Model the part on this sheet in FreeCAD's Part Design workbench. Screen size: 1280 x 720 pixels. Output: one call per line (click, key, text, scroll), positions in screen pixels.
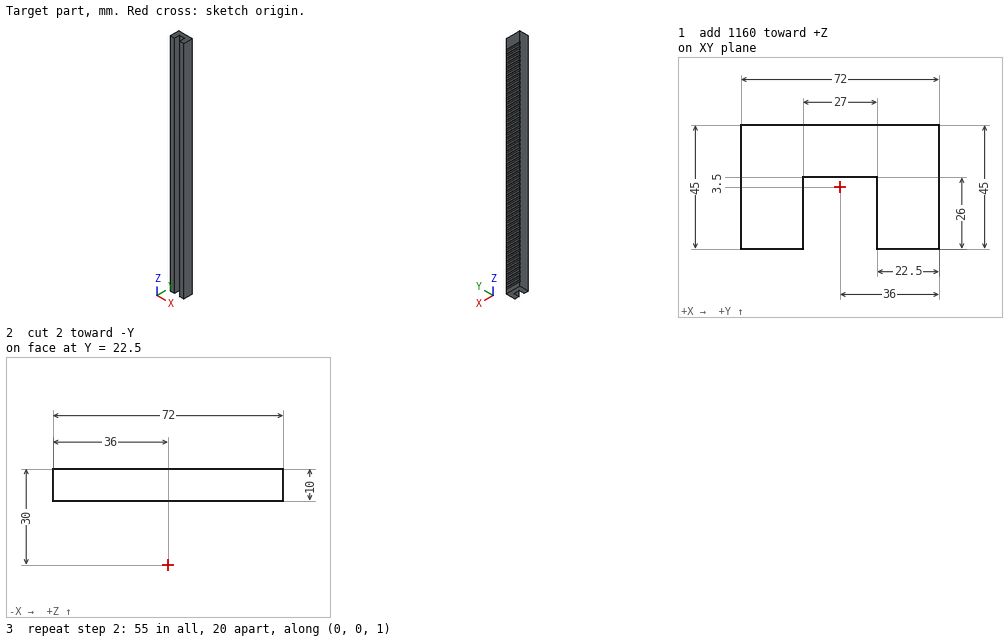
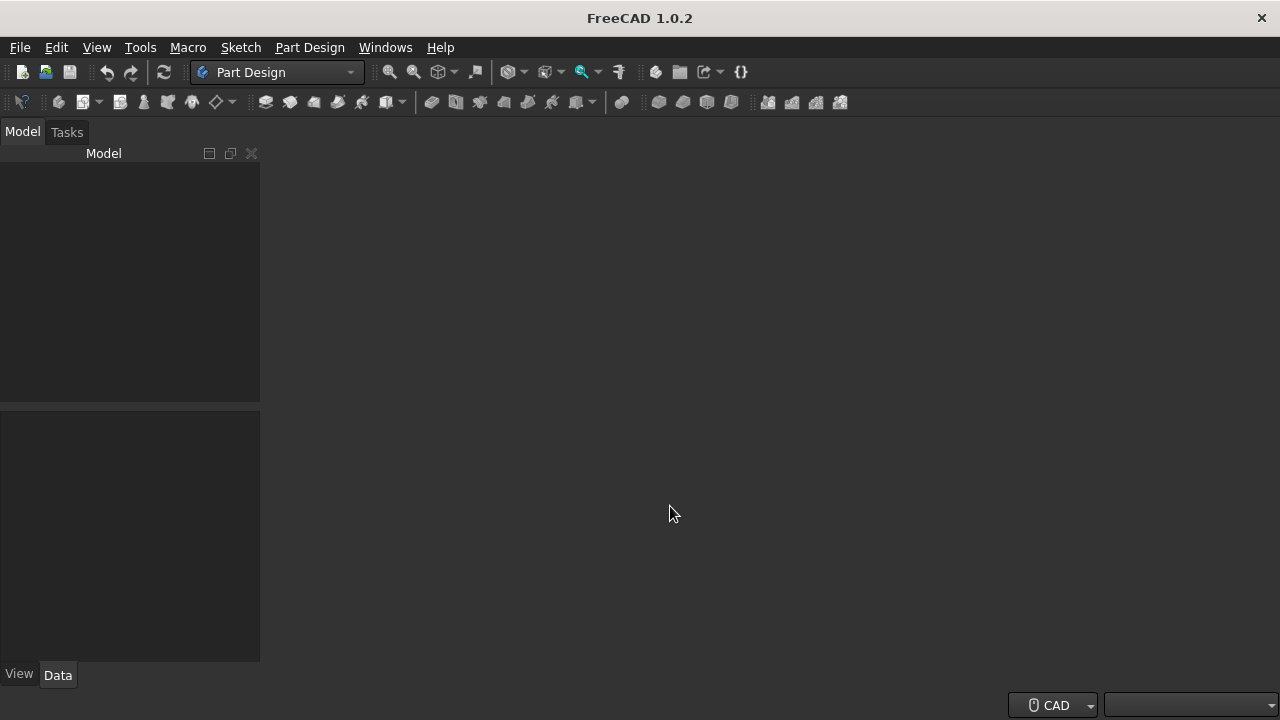
key(ctrl+n)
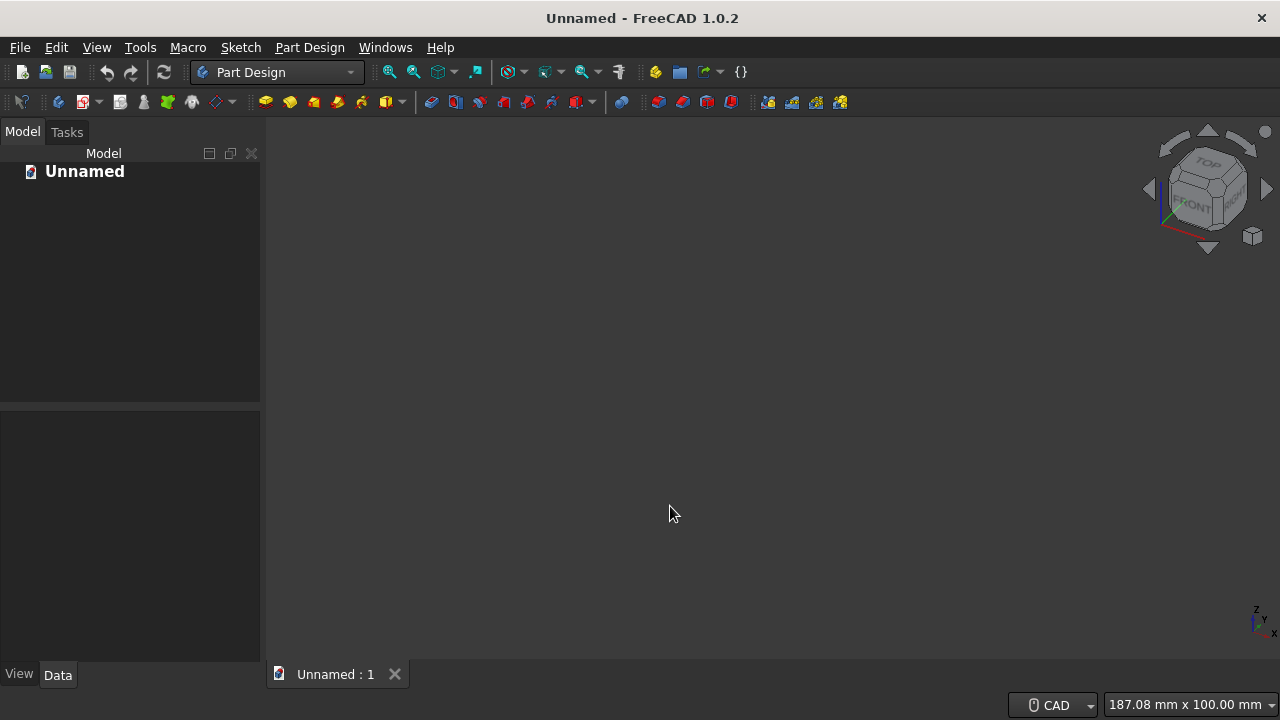
click(84, 102)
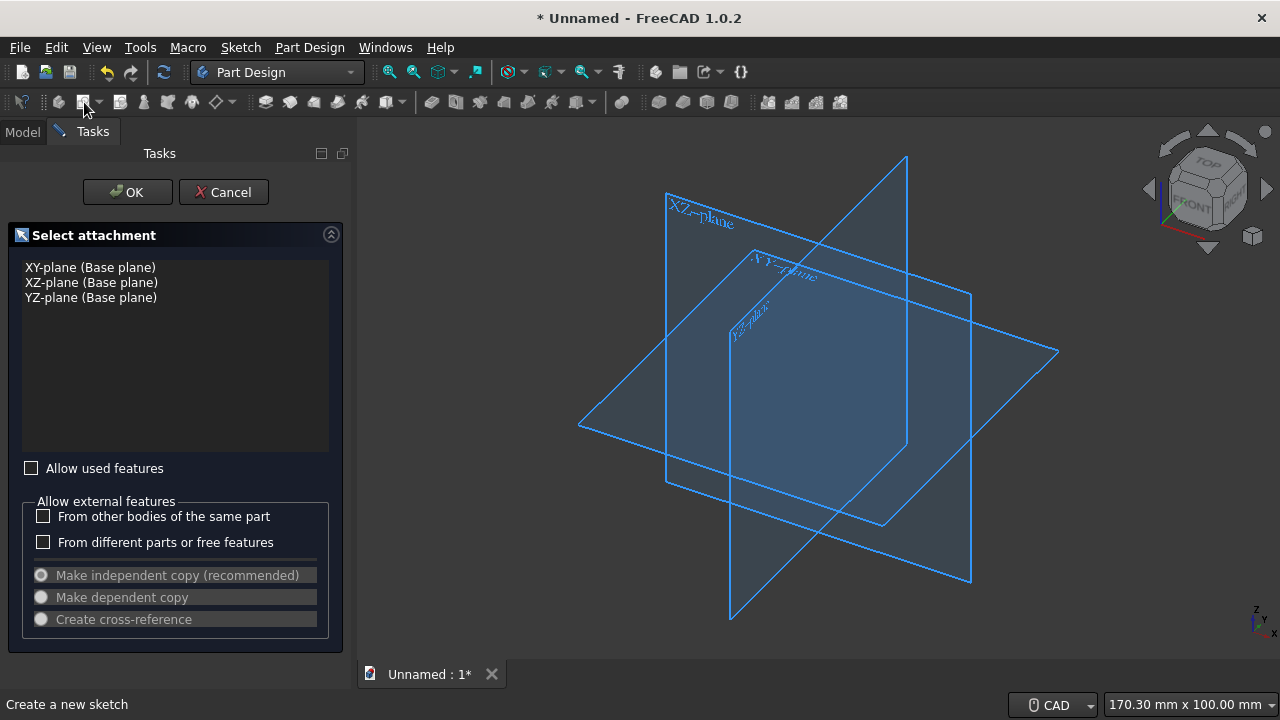
click(82, 268)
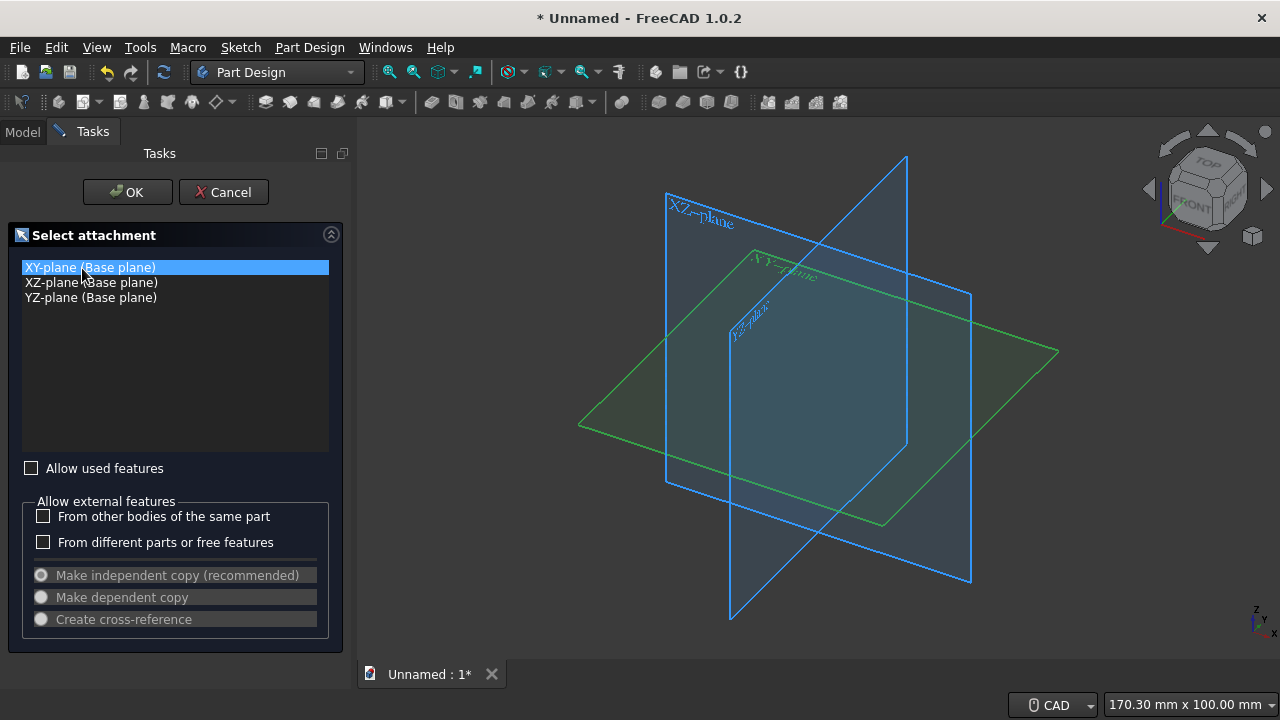
click(128, 192)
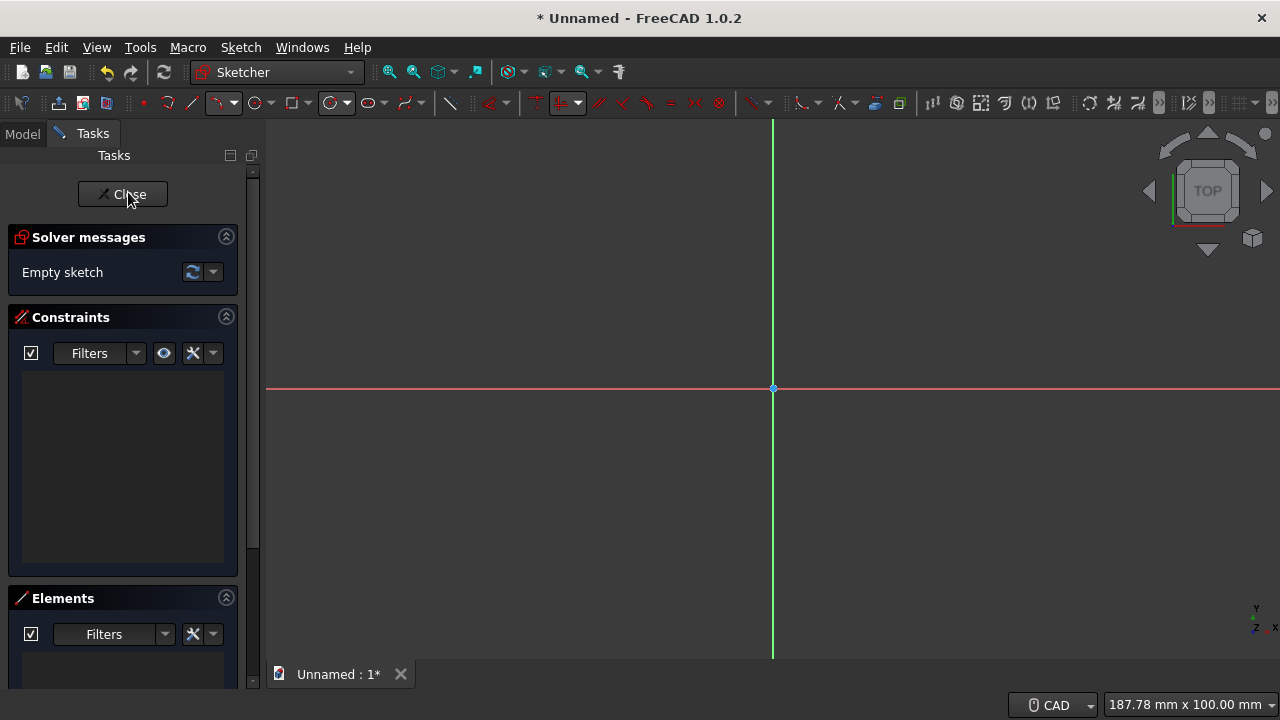
scroll(912, 389, up, 2)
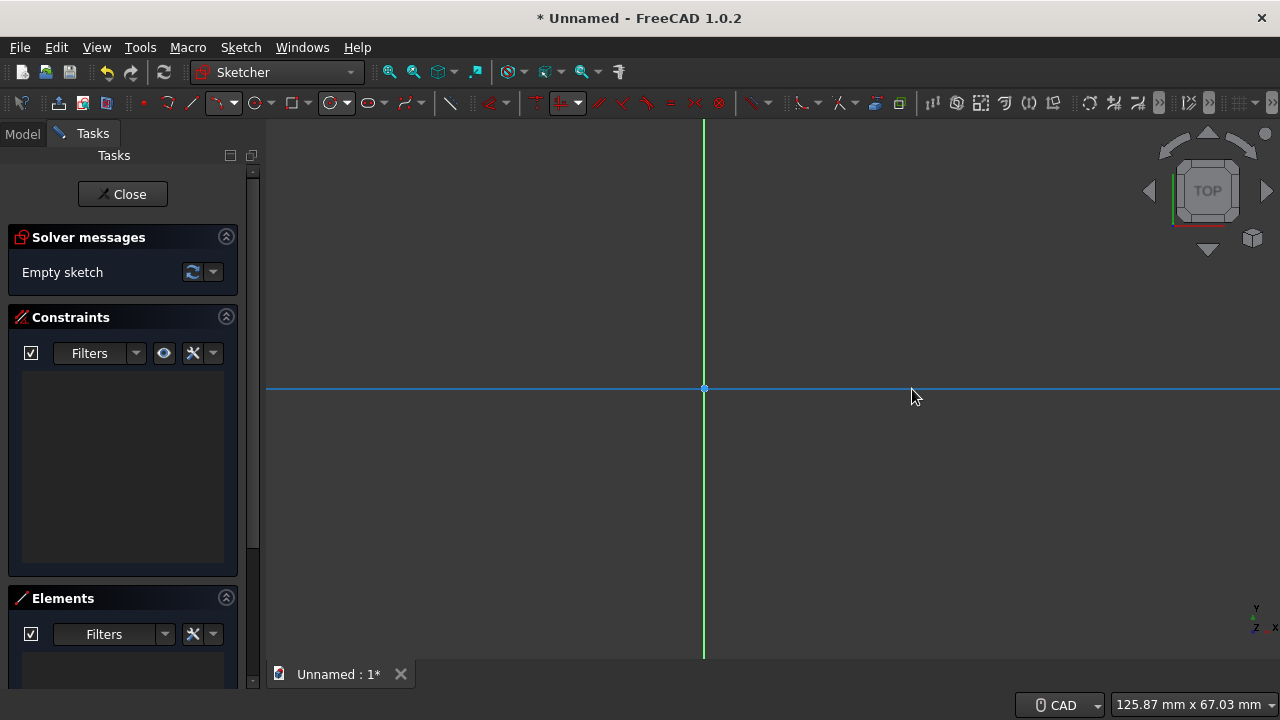
key(g)
key(m)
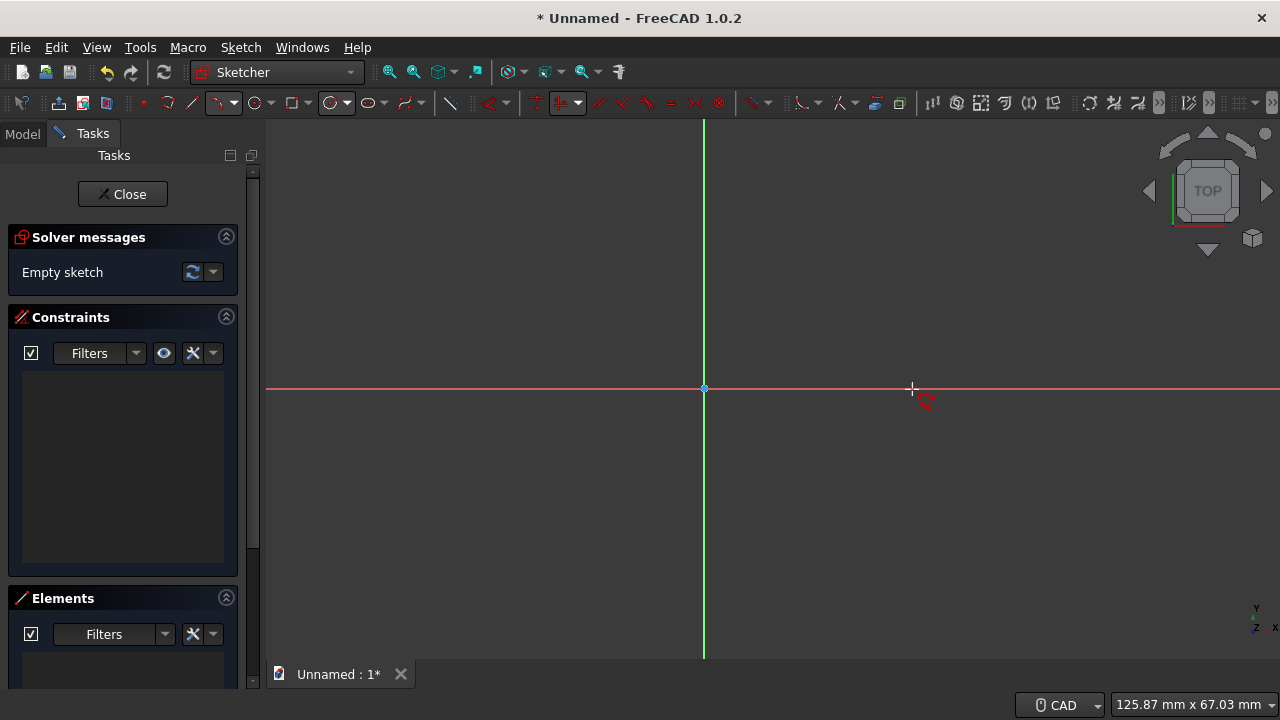
click(596, 361)
click(813, 361)
click(813, 570)
click(994, 570)
click(994, 207)
click(414, 207)
click(414, 570)
click(596, 570)
click(596, 362)
key(Escape)
key(Escape)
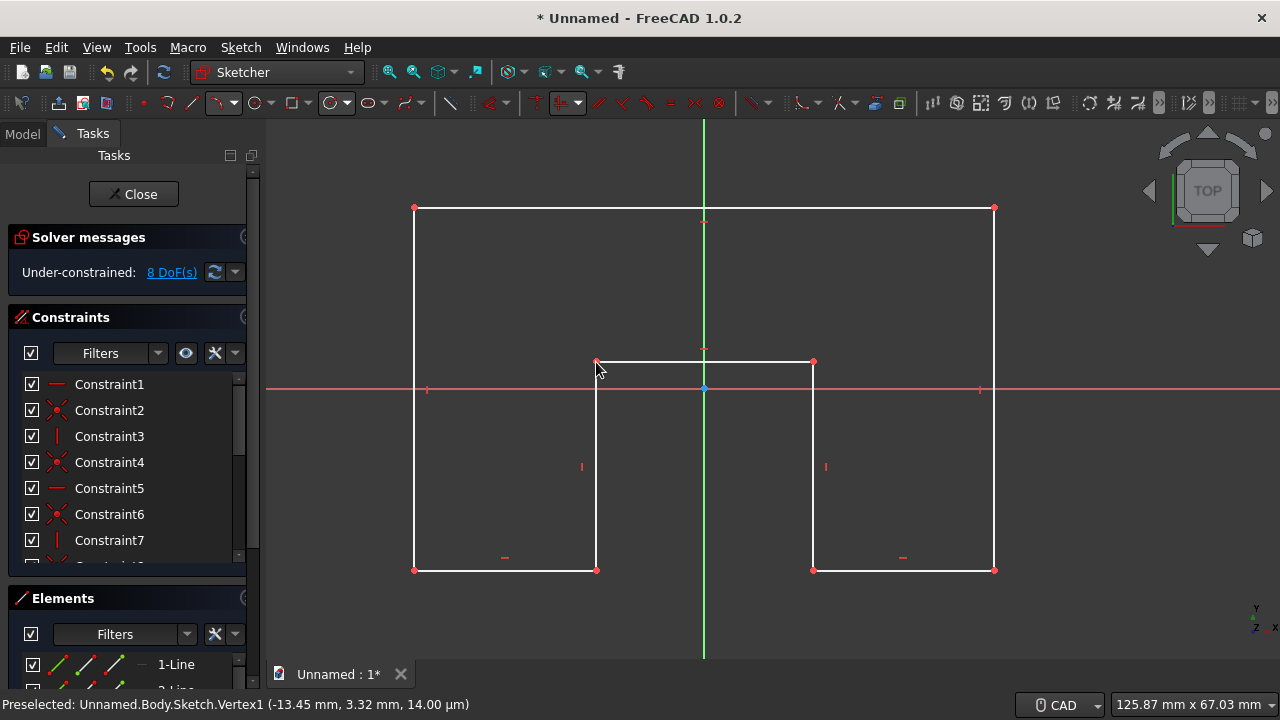
click(490, 104)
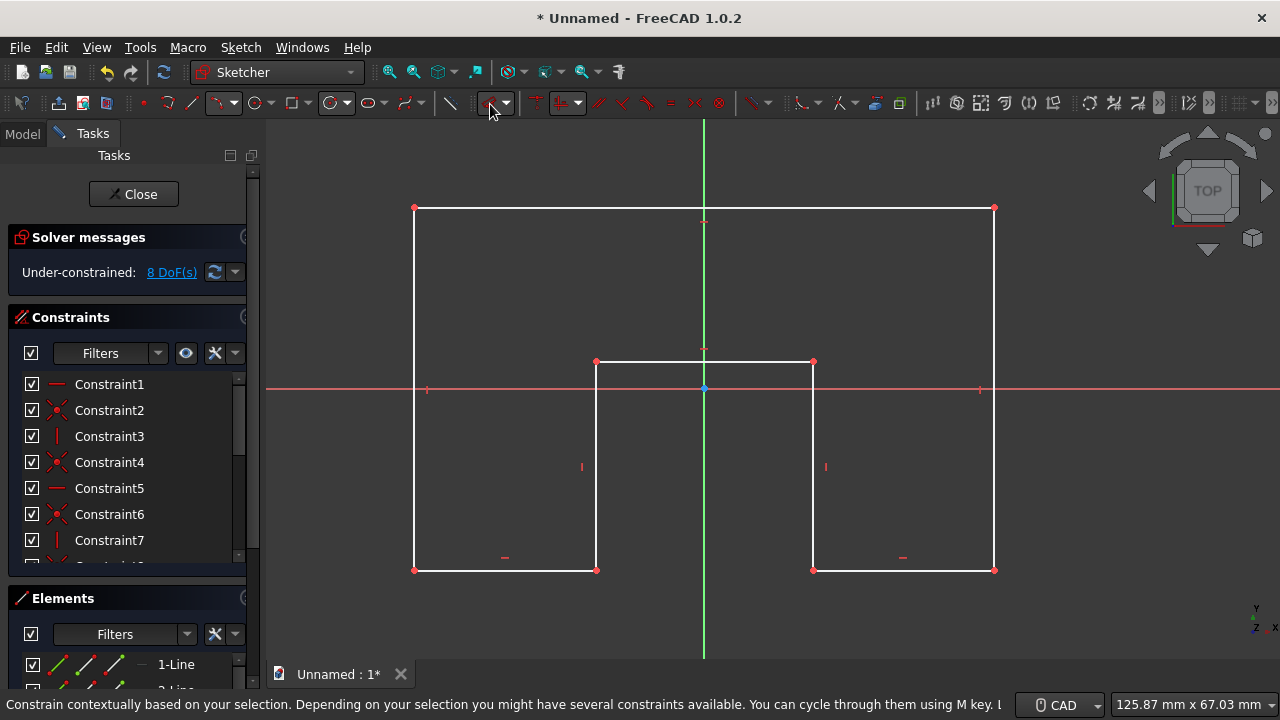
click(661, 362)
click(655, 328)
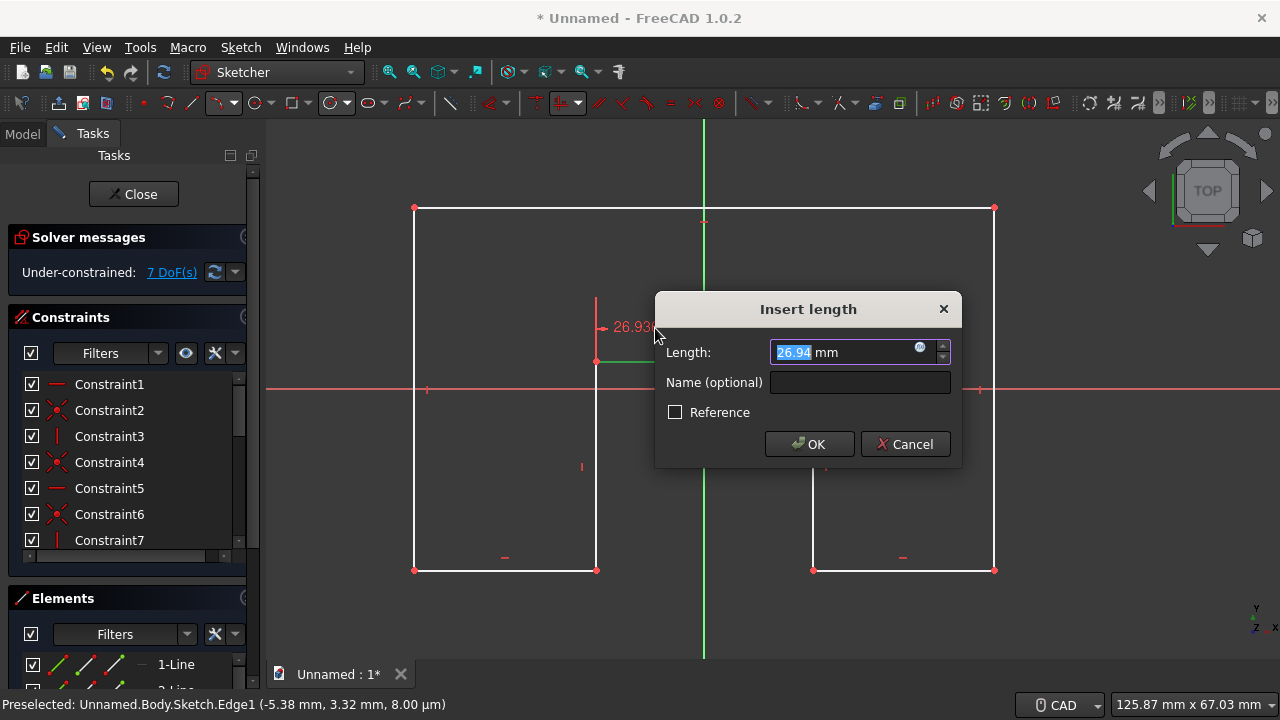
text(27)
key(Return)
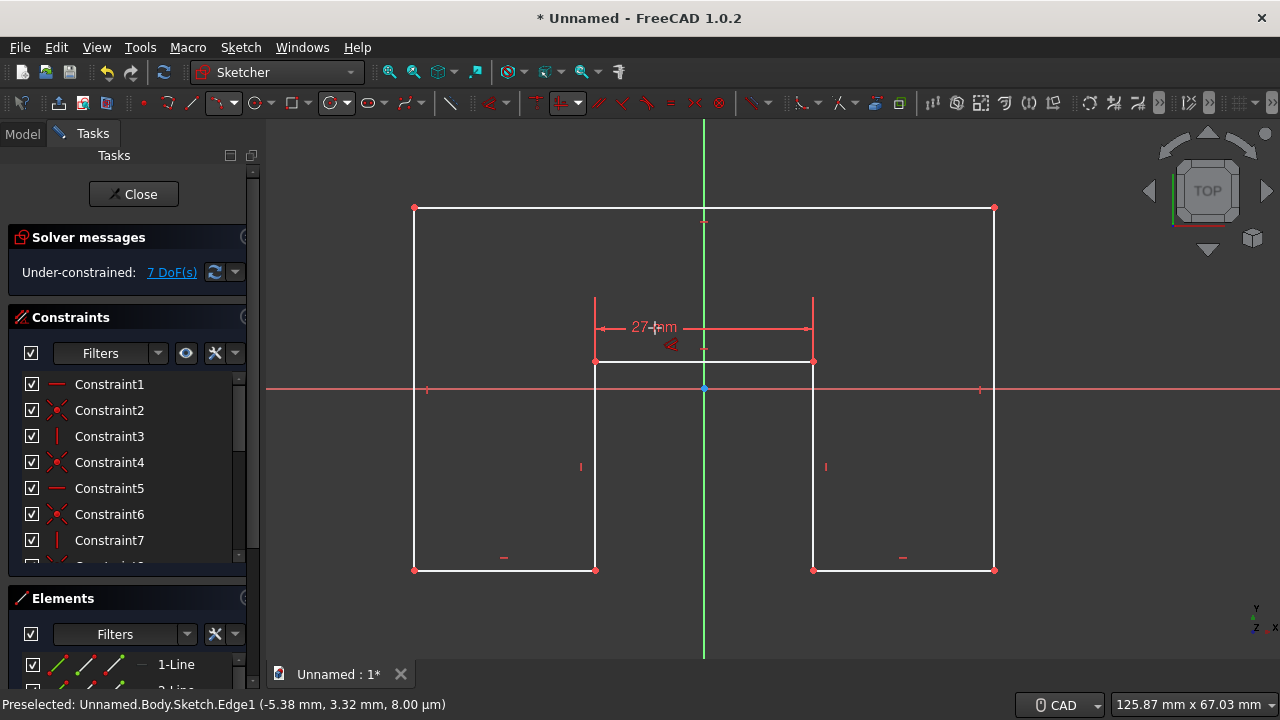
click(813, 425)
click(847, 466)